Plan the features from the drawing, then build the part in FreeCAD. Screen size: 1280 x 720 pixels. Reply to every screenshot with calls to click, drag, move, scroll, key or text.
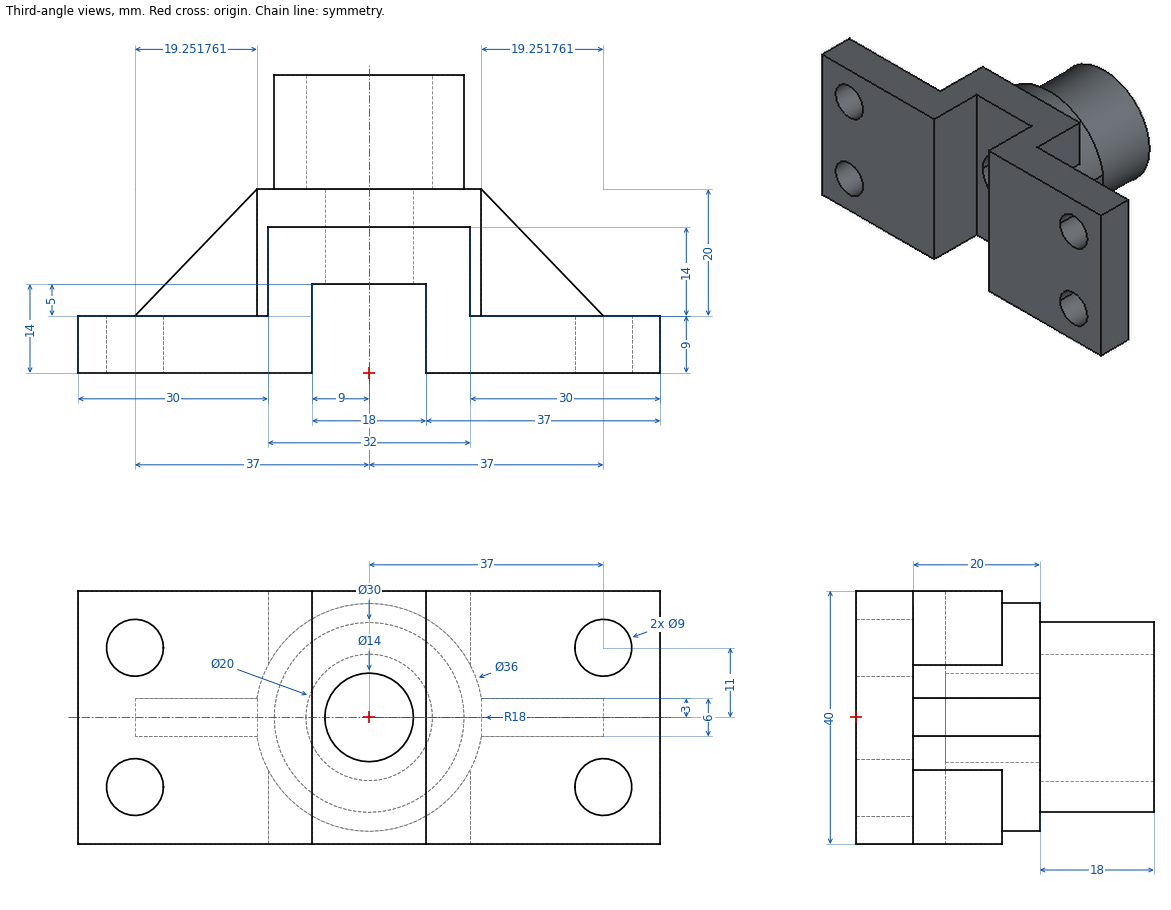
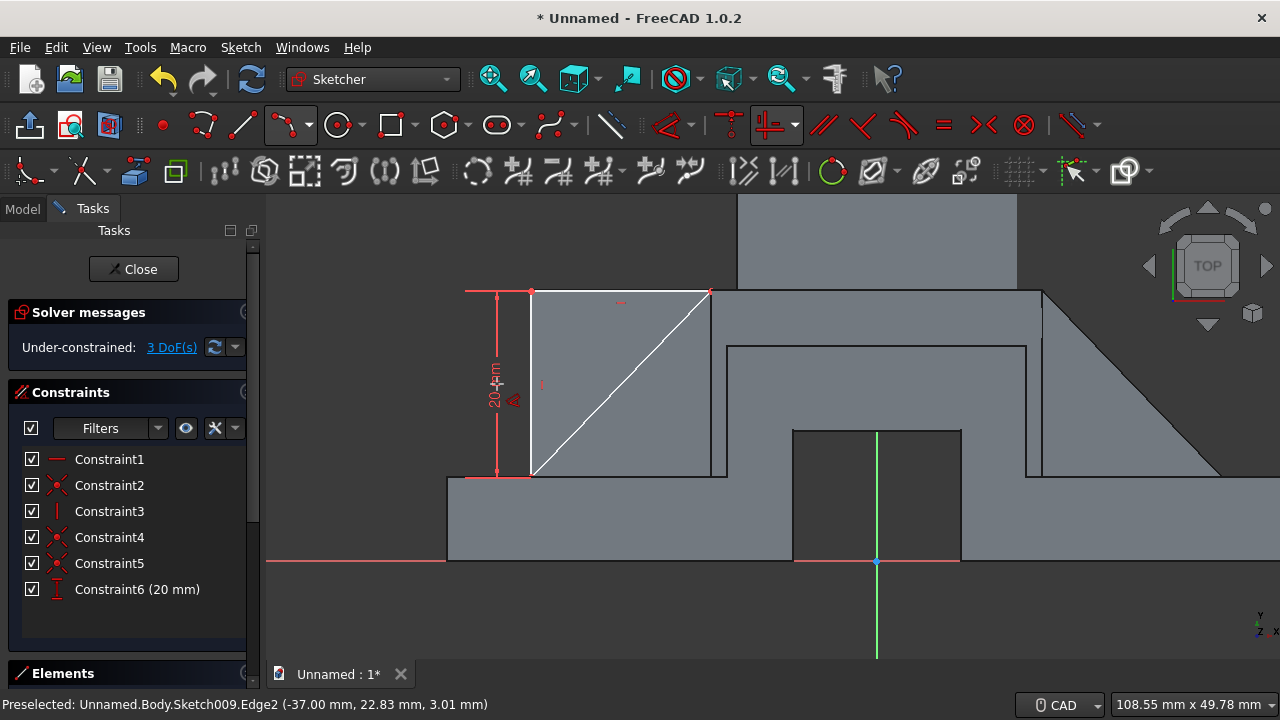
click(531, 478)
click(497, 520)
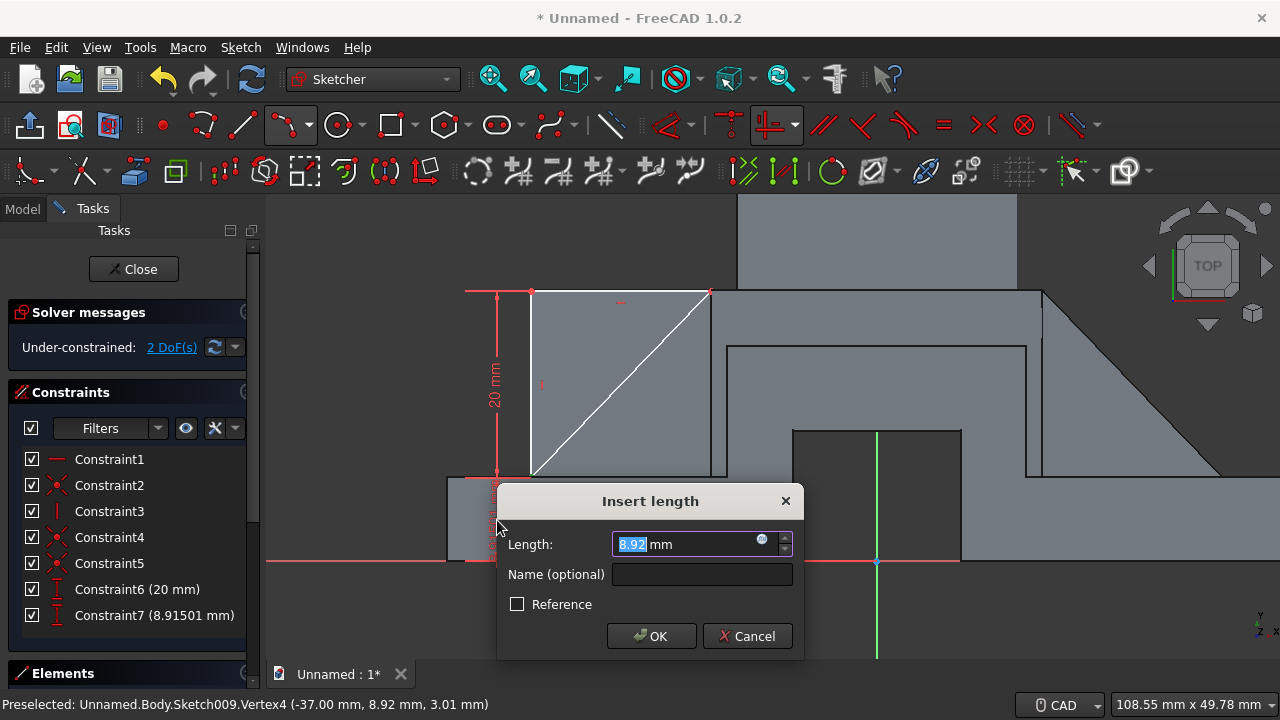
text(9)
key(Return)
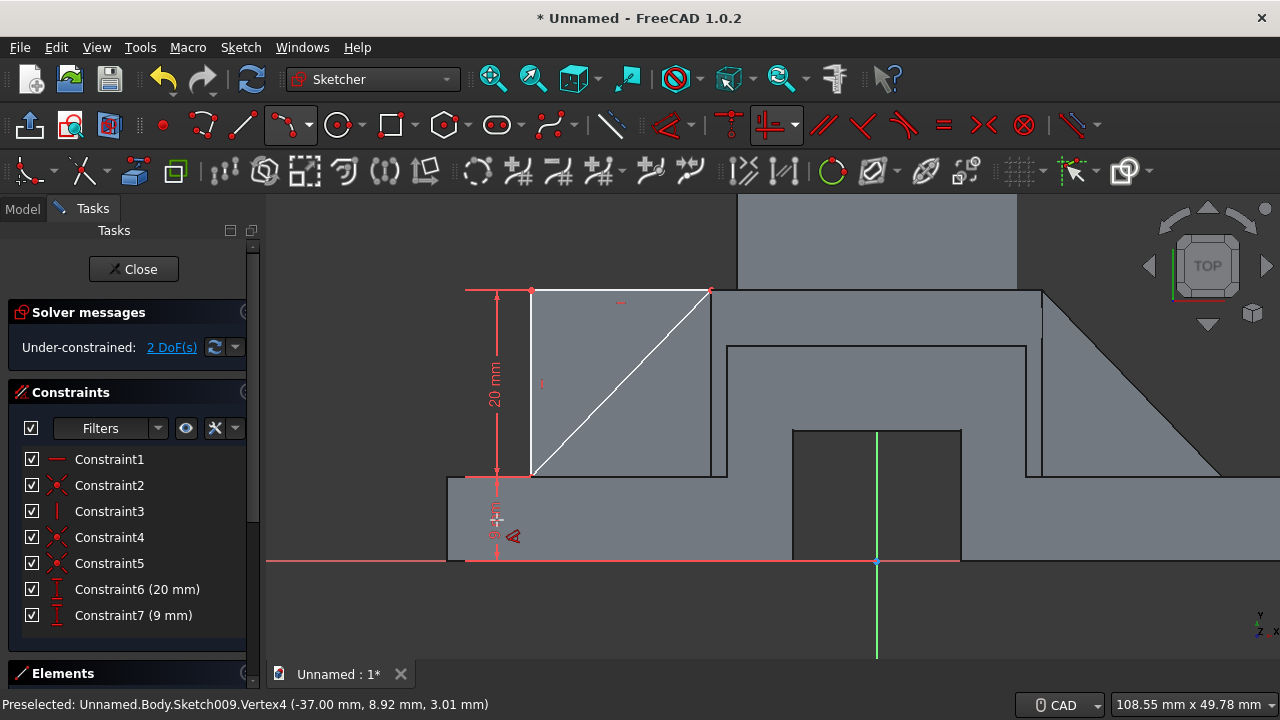
click(531, 290)
click(704, 595)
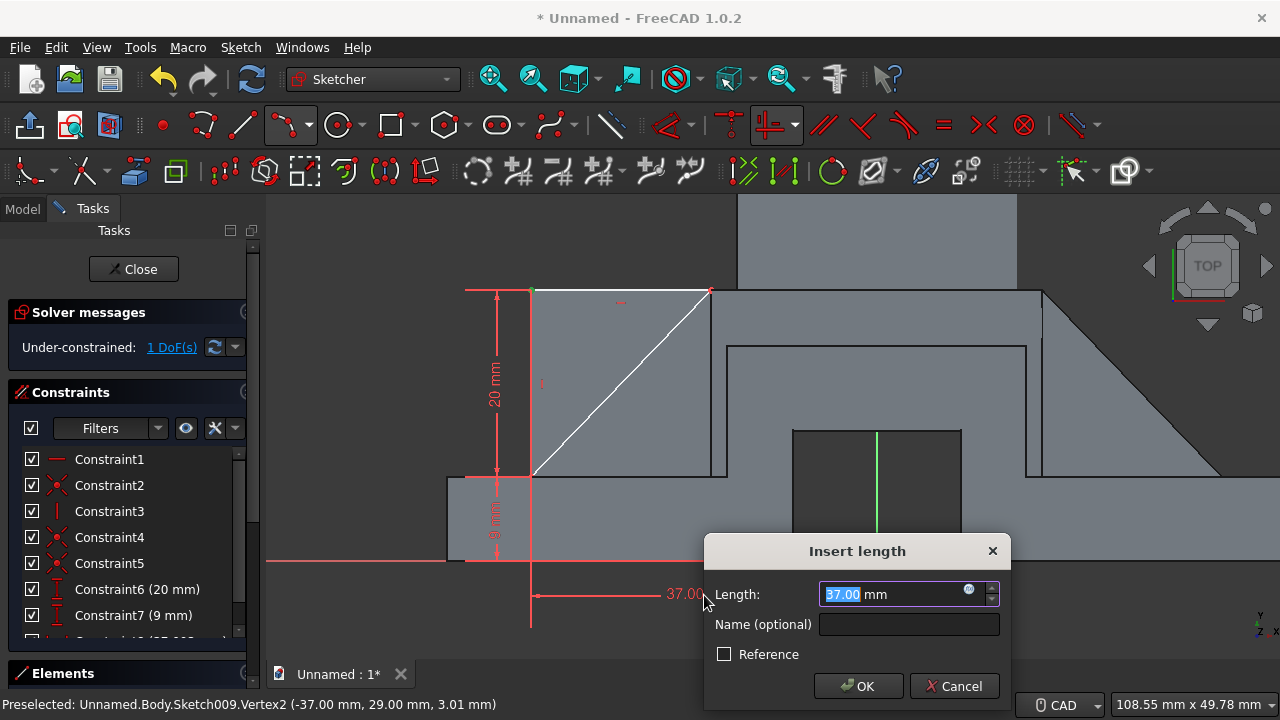
text(37)
key(Return)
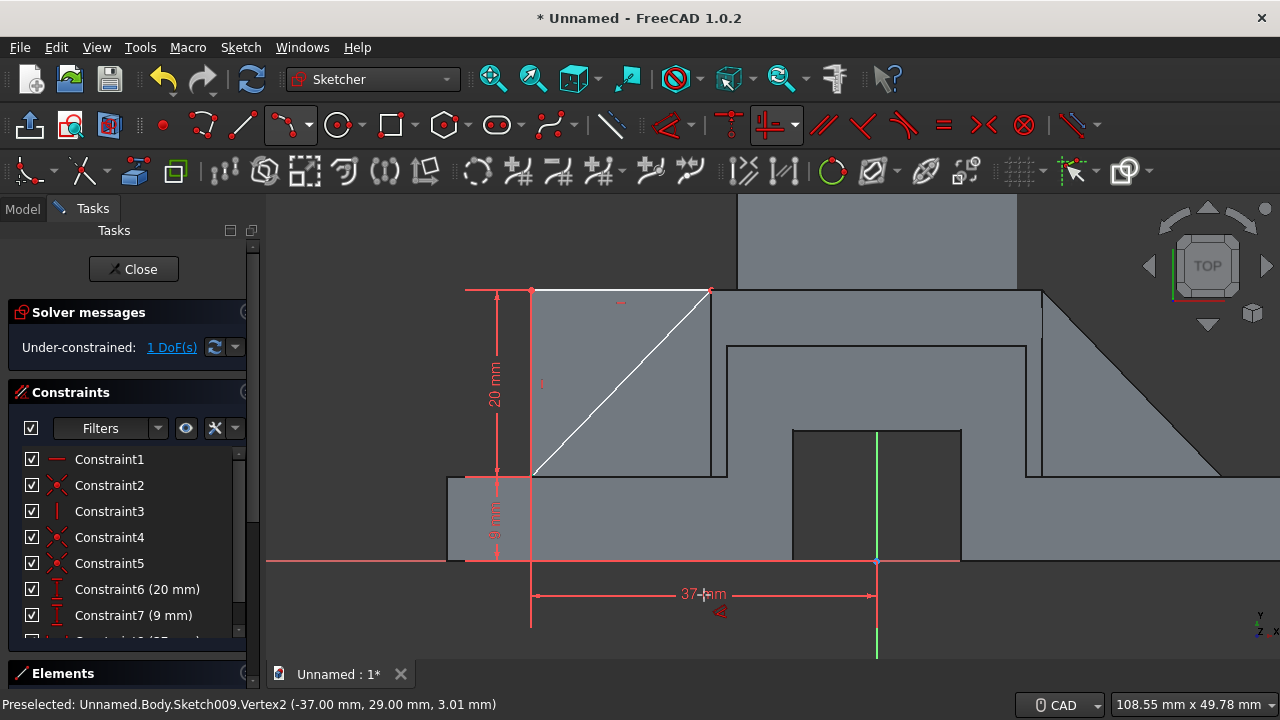
click(657, 290)
click(621, 256)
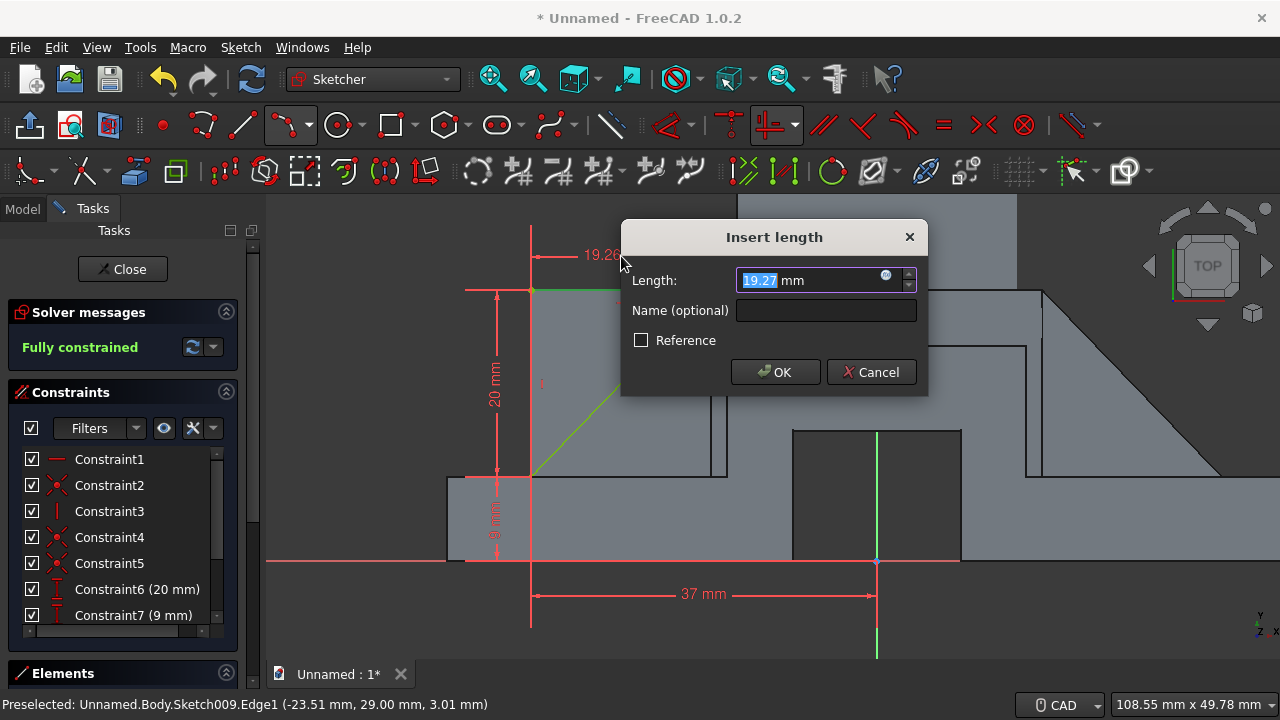
text(19.251761)
key(Return)
key(Escape)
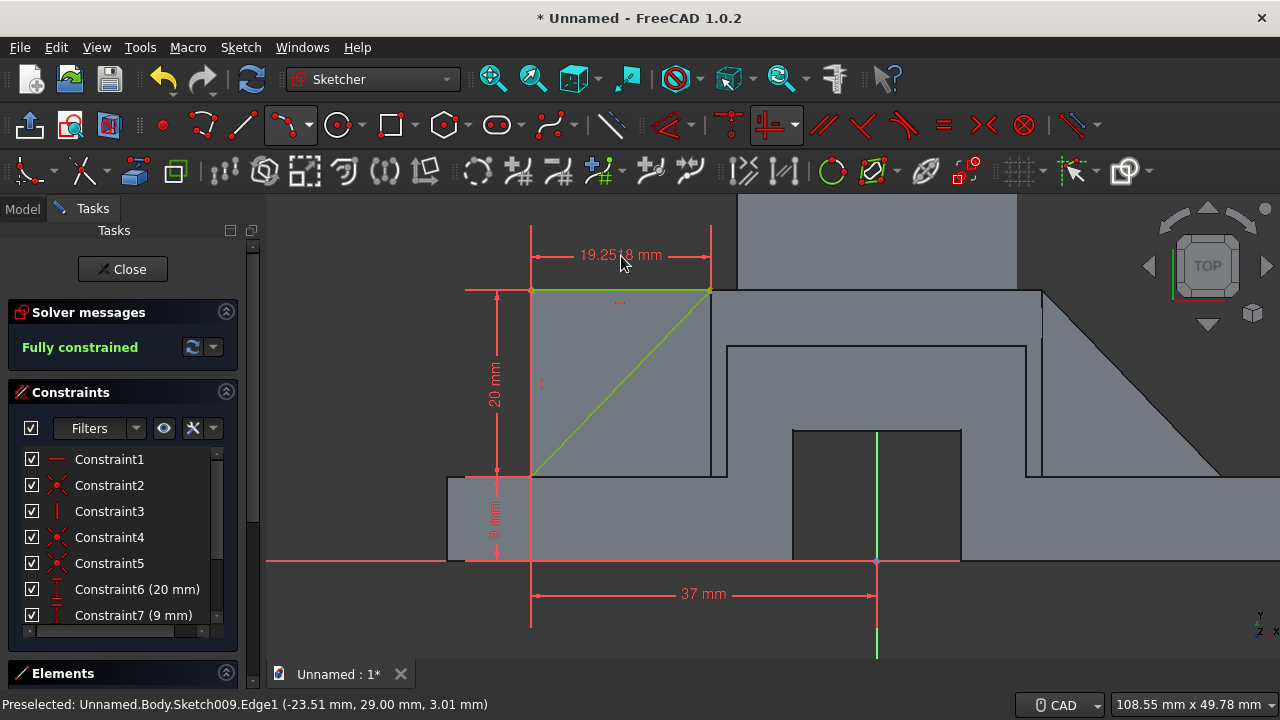
click(123, 269)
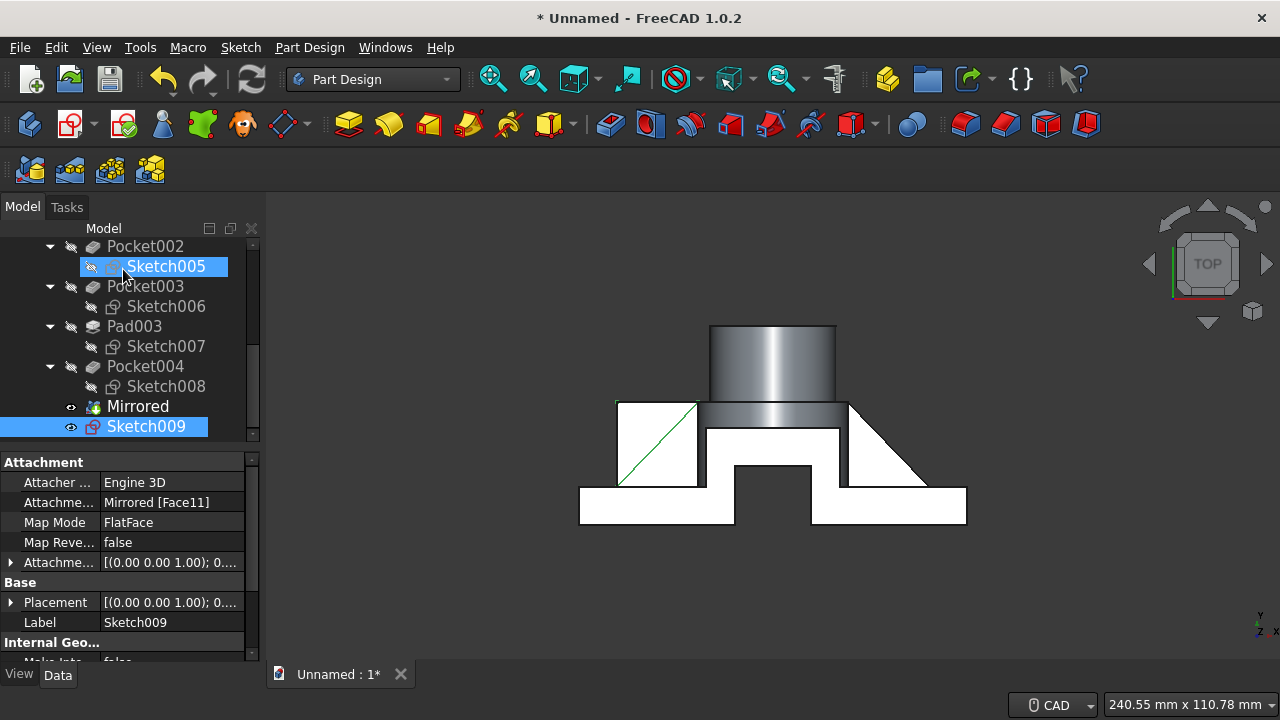
click(612, 124)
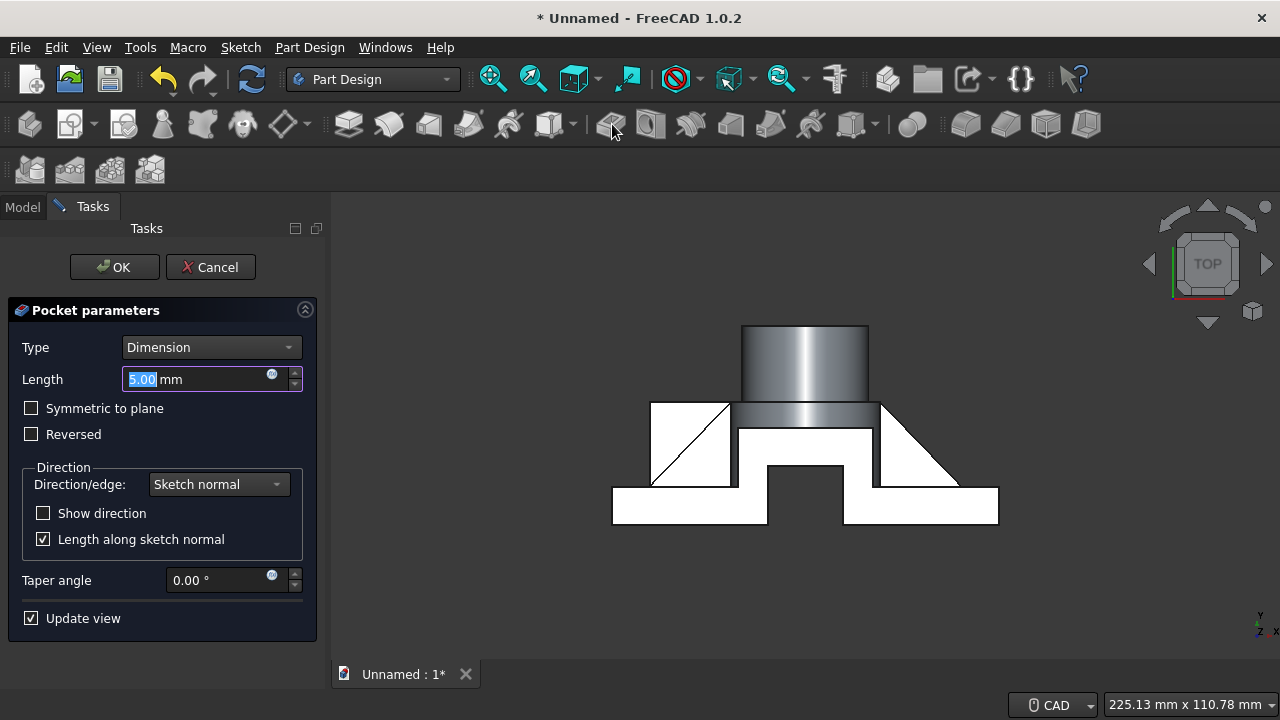
click(212, 348)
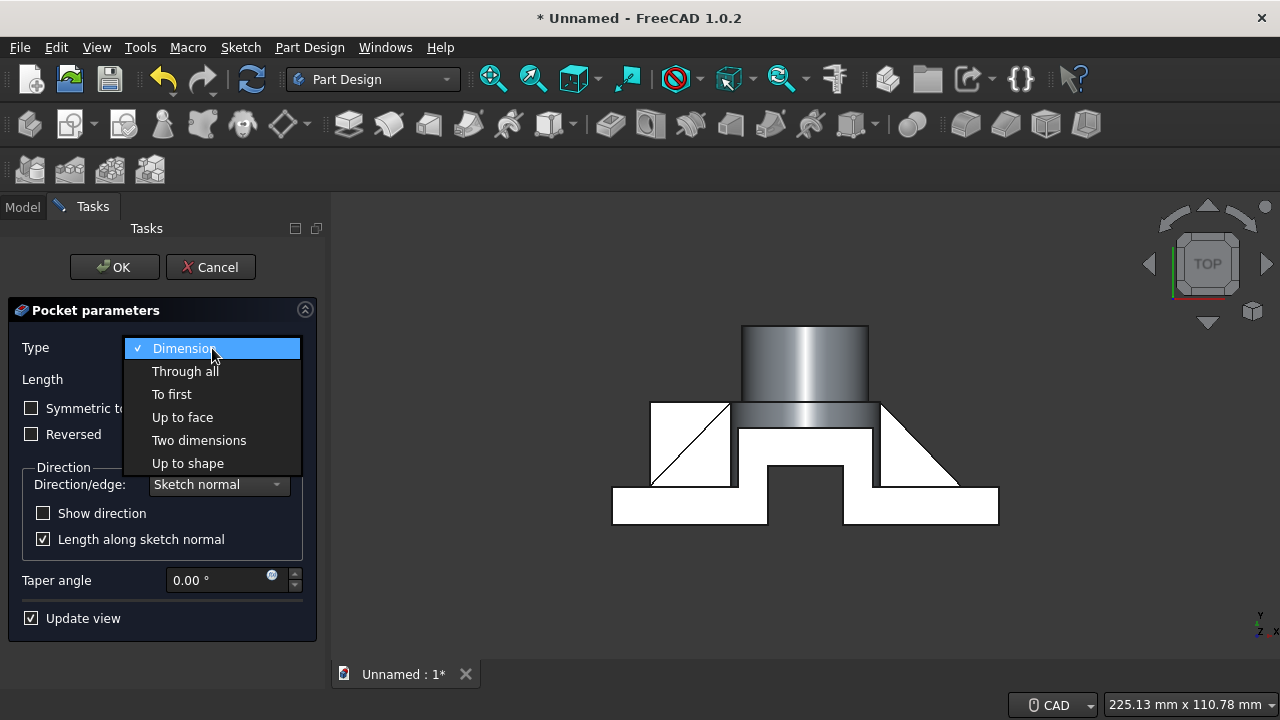
click(212, 372)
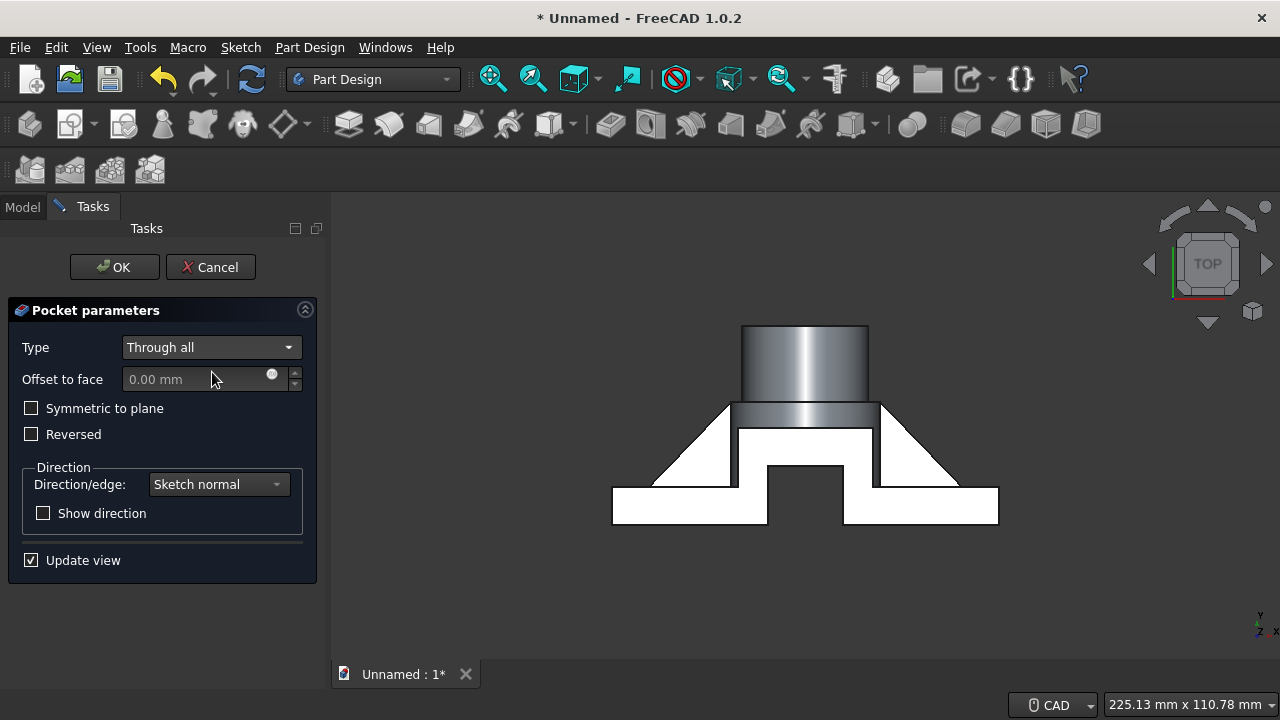
click(115, 267)